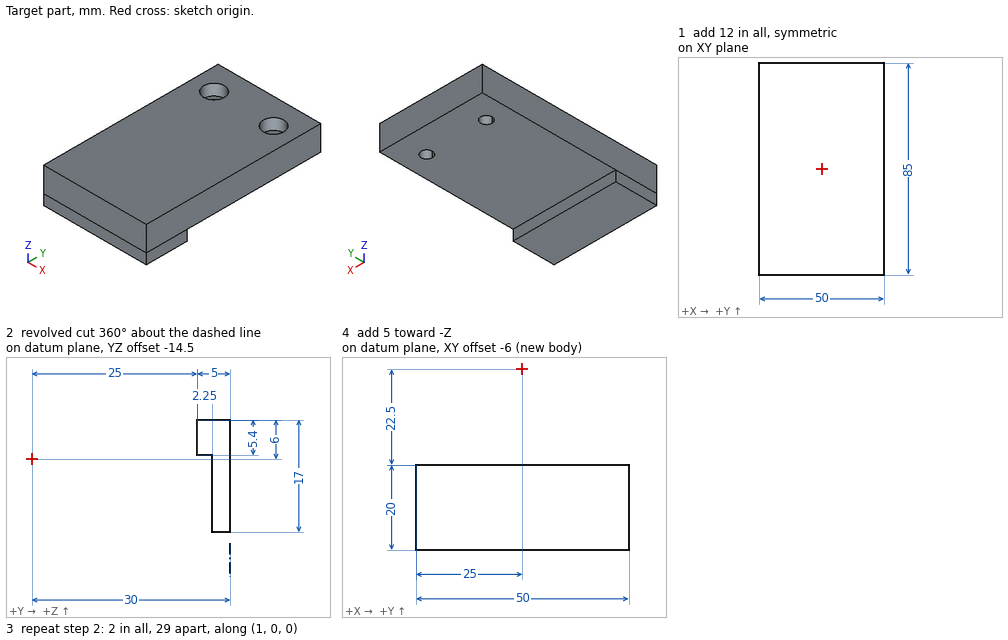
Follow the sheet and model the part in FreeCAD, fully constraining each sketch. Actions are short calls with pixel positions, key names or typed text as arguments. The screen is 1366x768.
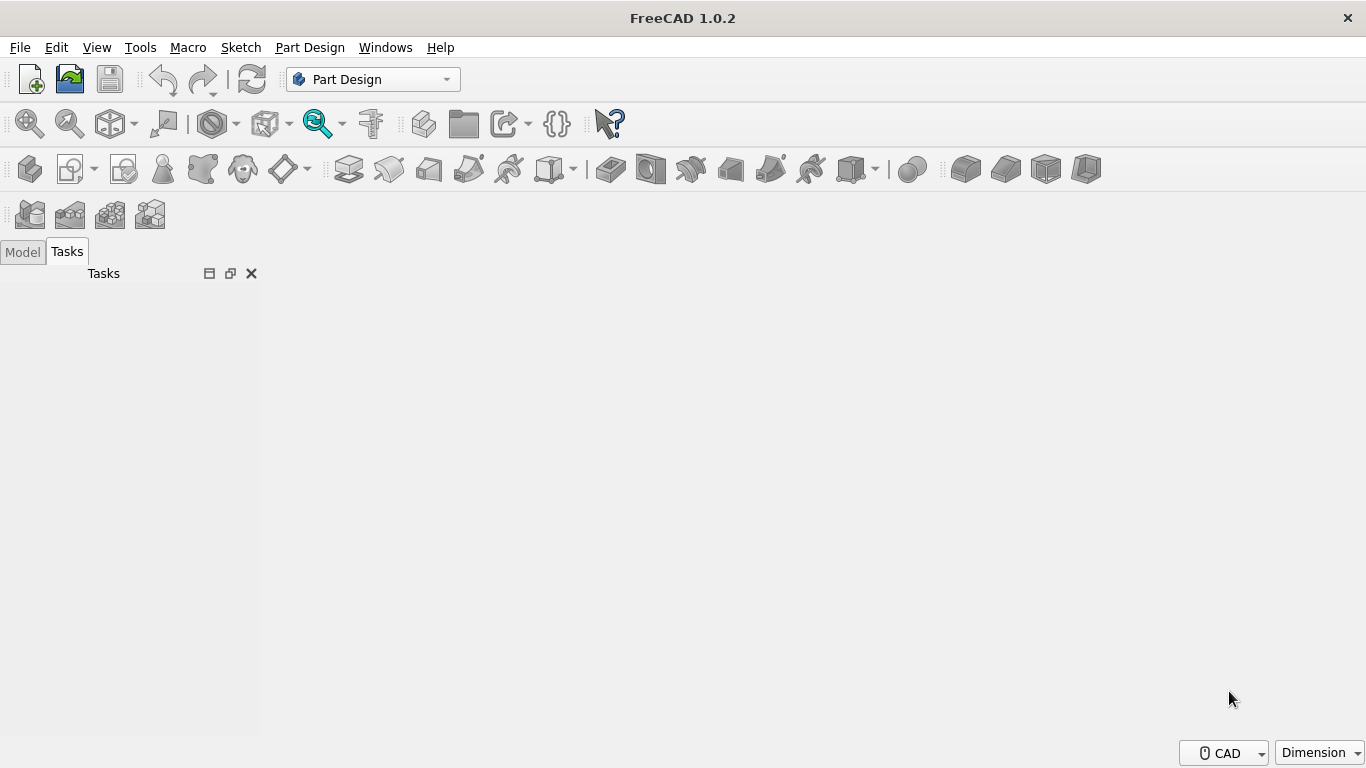
key(ctrl+n)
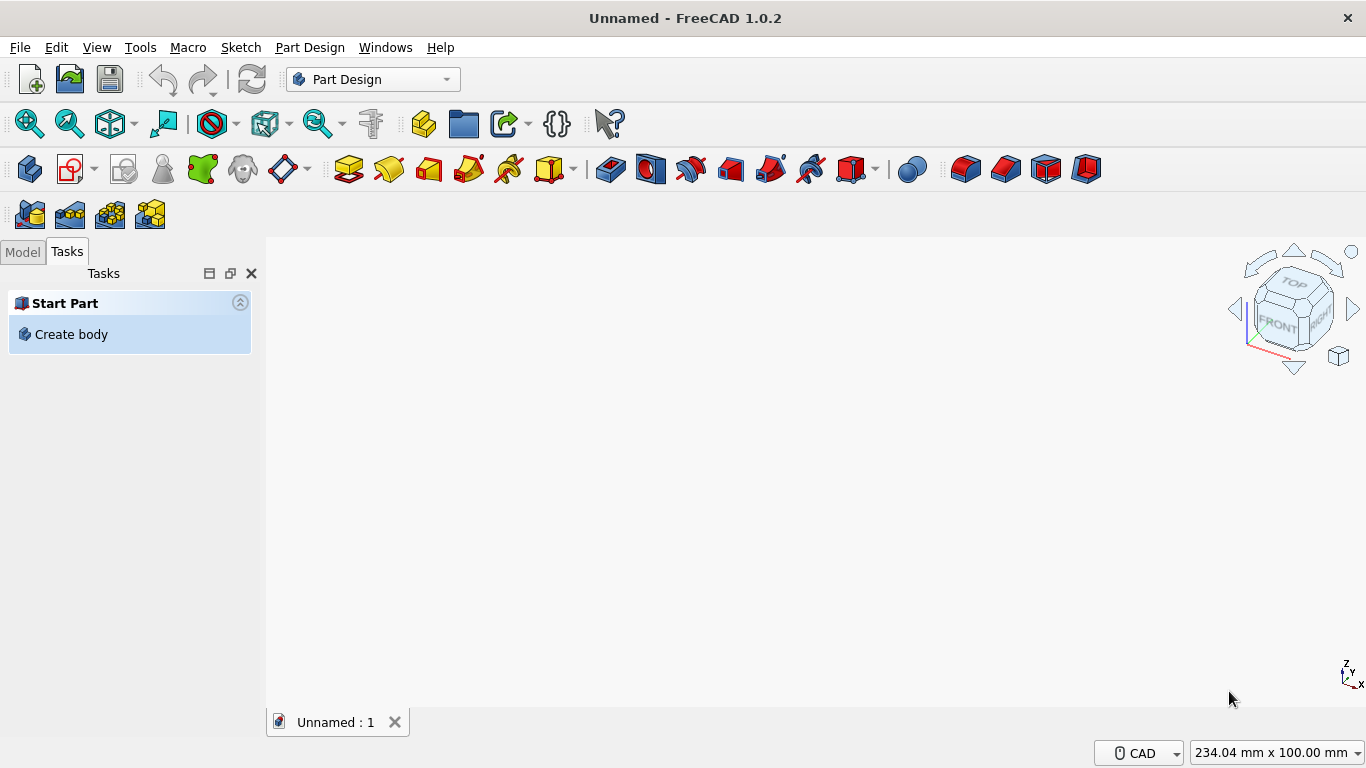
click(70, 170)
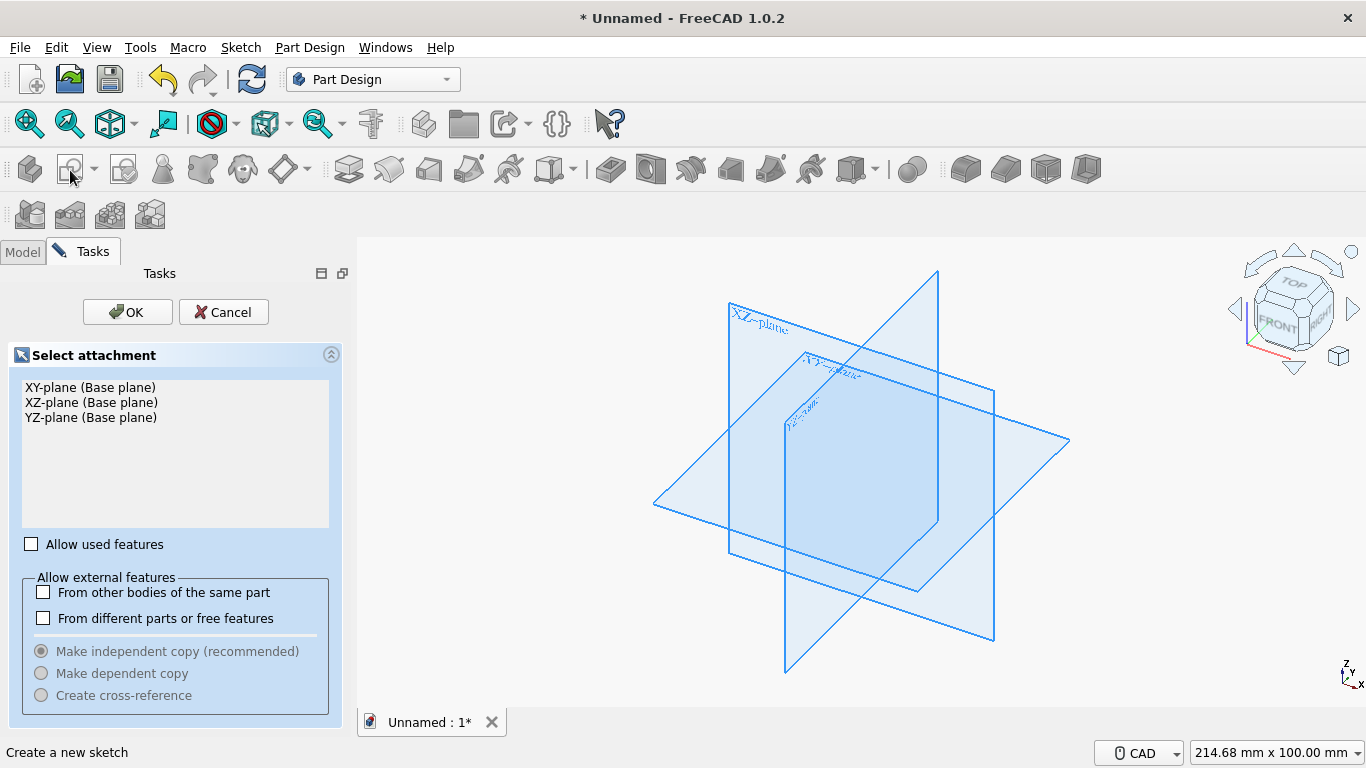
click(82, 388)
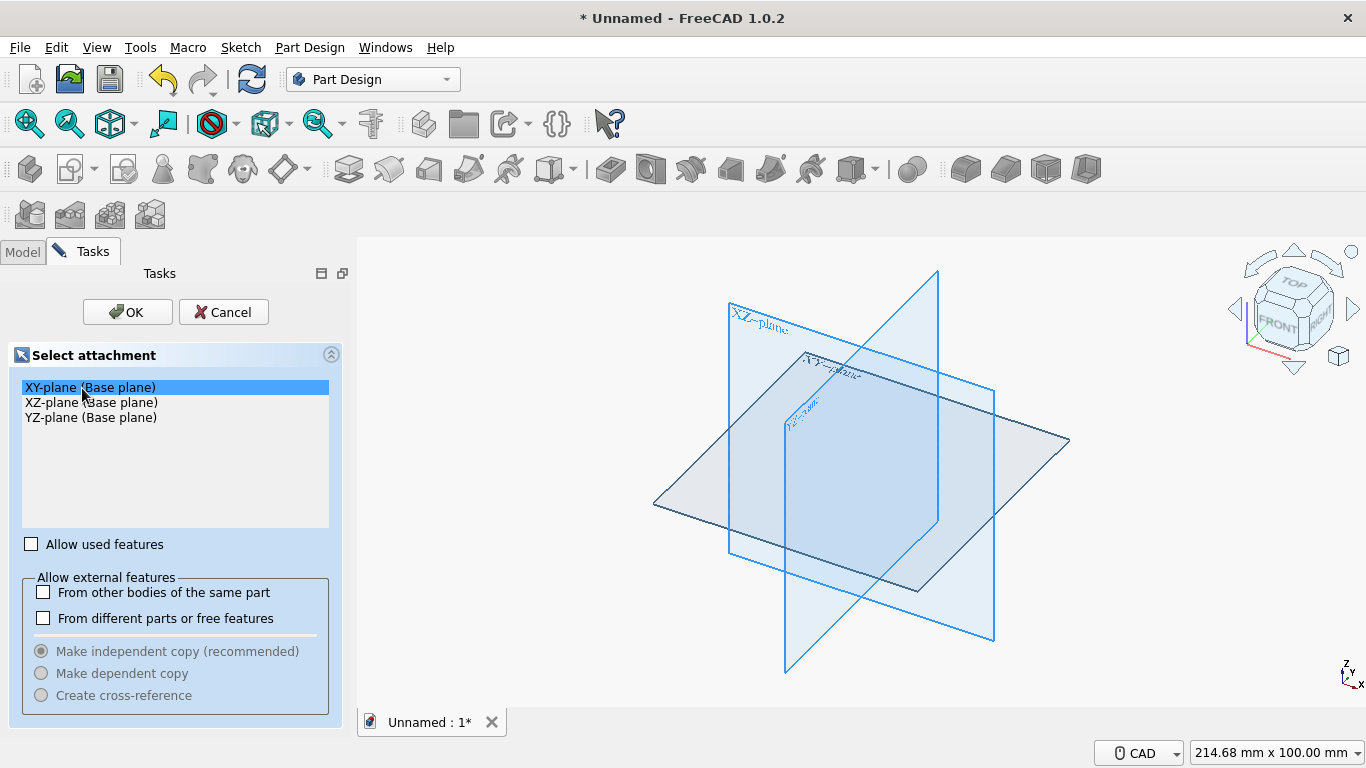
click(128, 312)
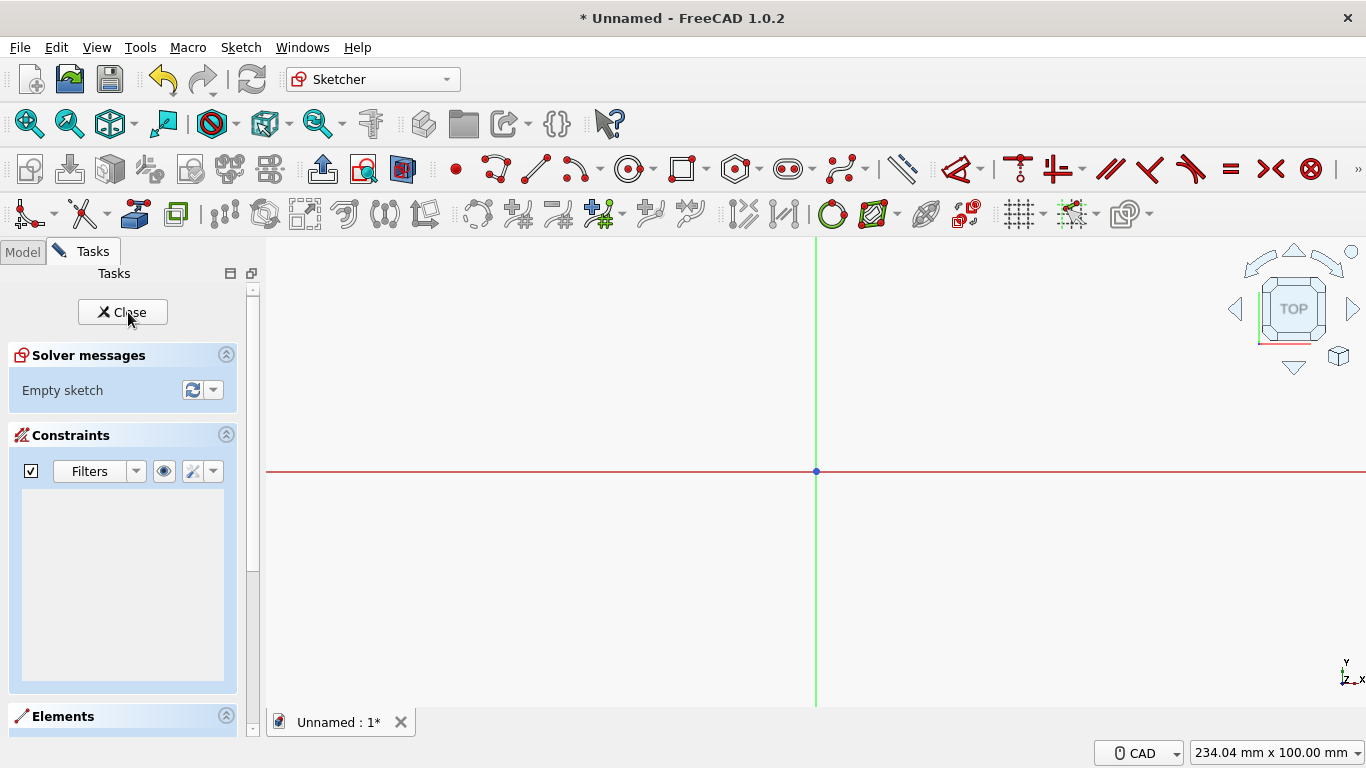
scroll(608, 472, down, 2)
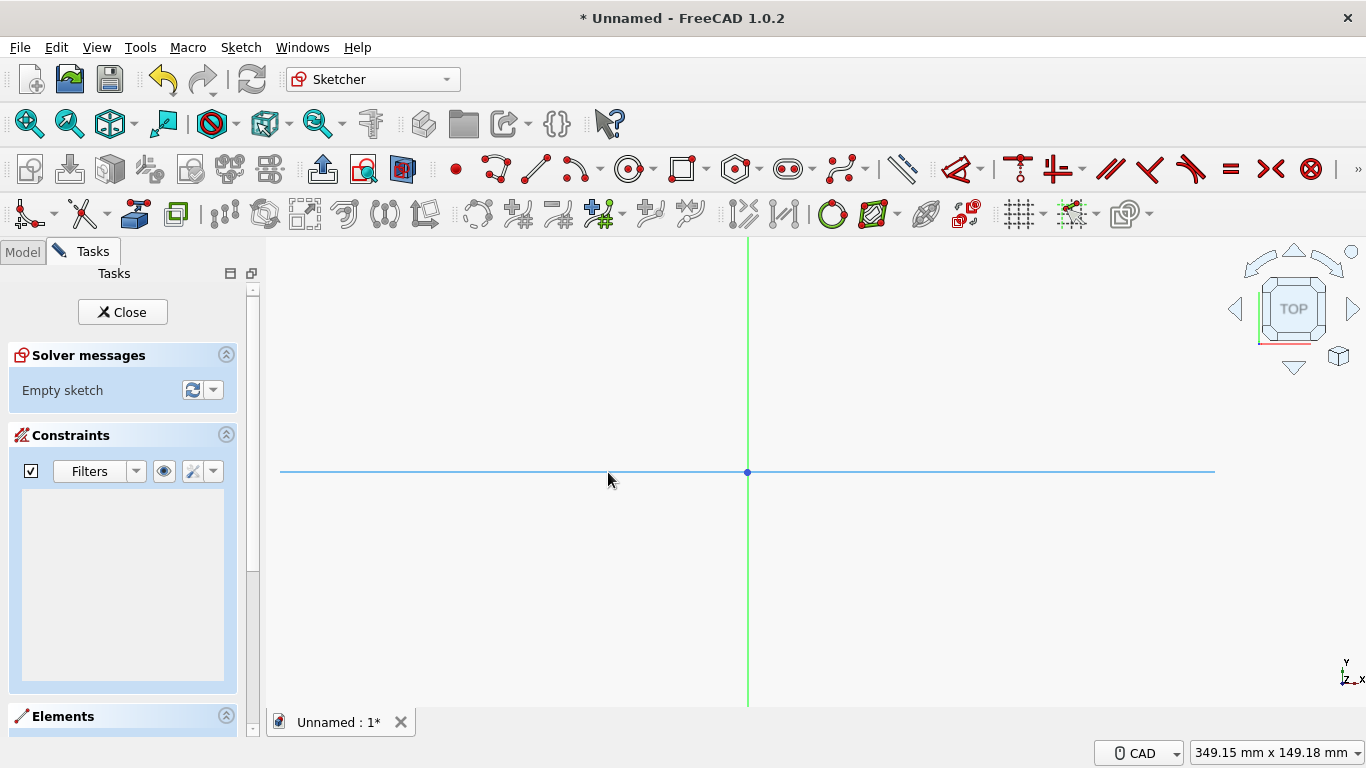
click(708, 170)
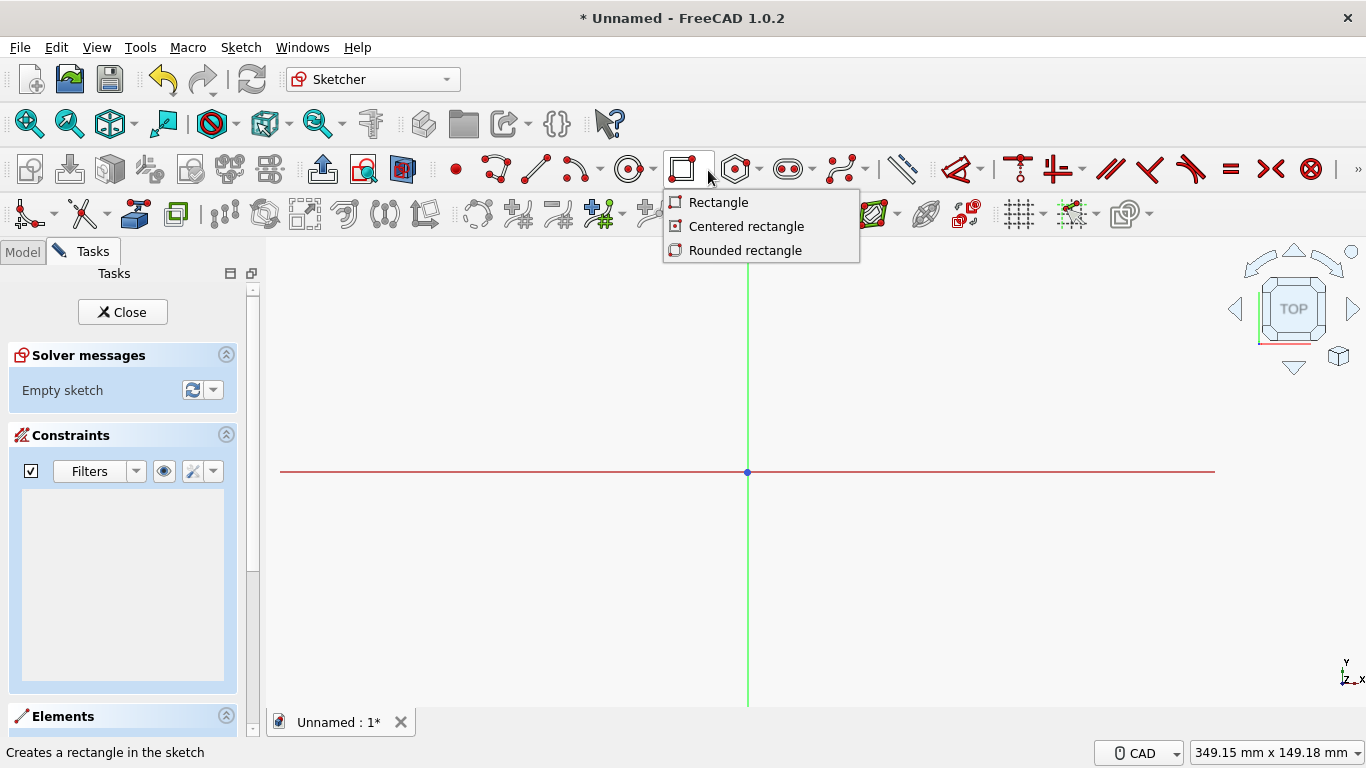
click(762, 226)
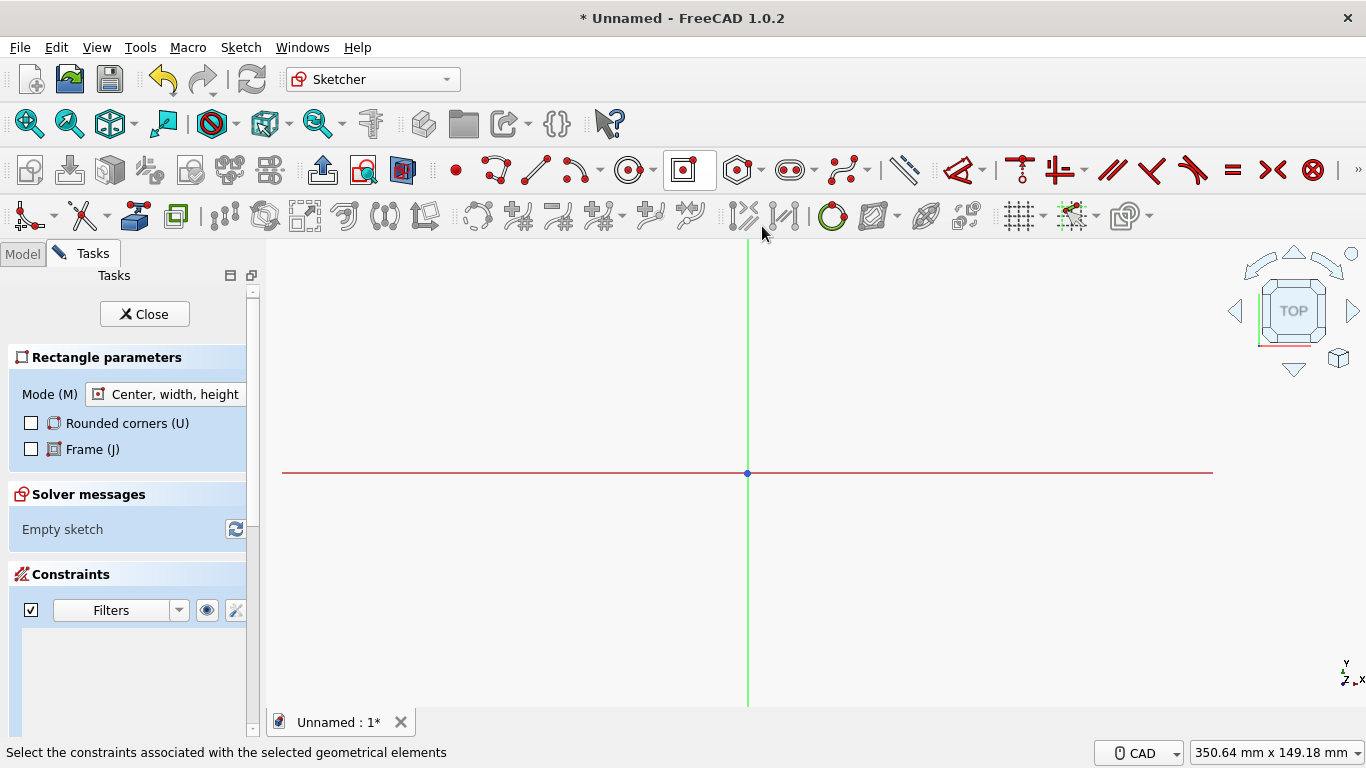
click(748, 473)
click(826, 340)
key(Escape)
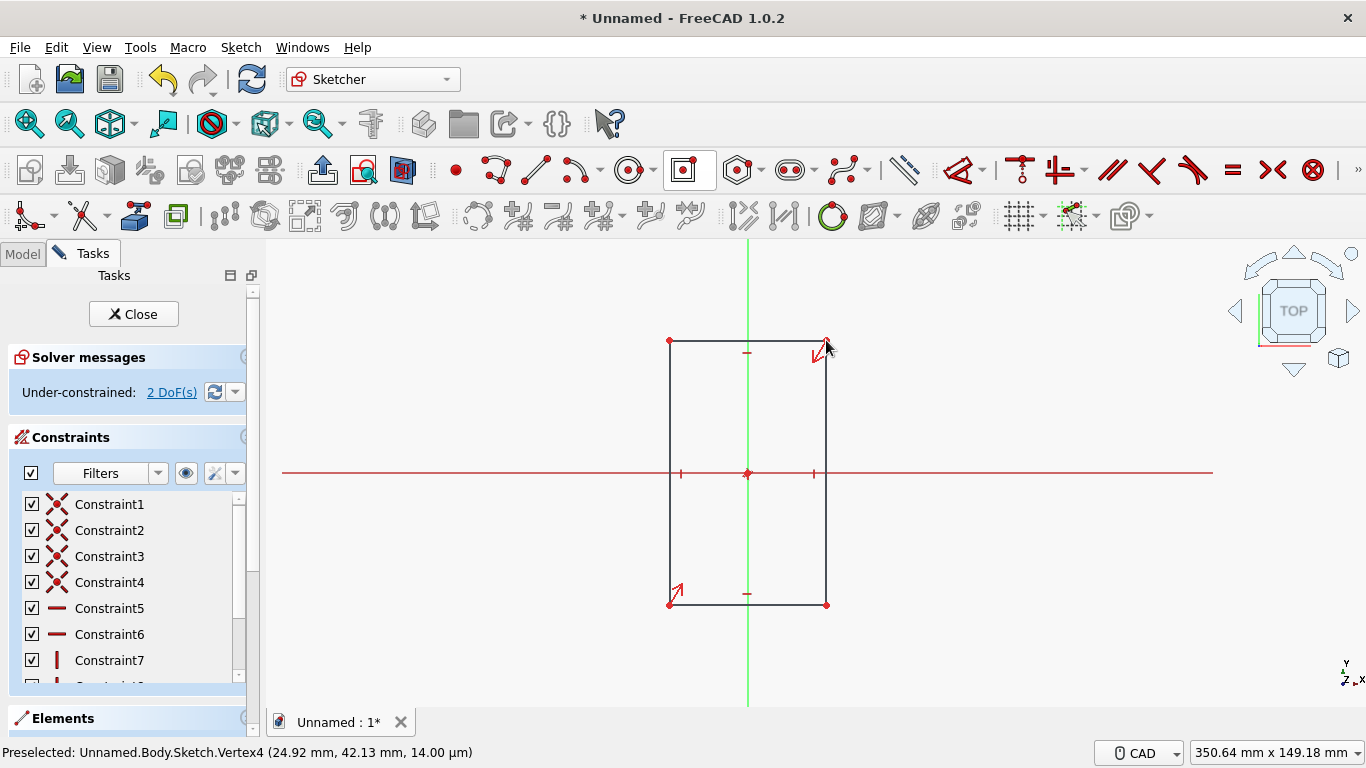
key(d)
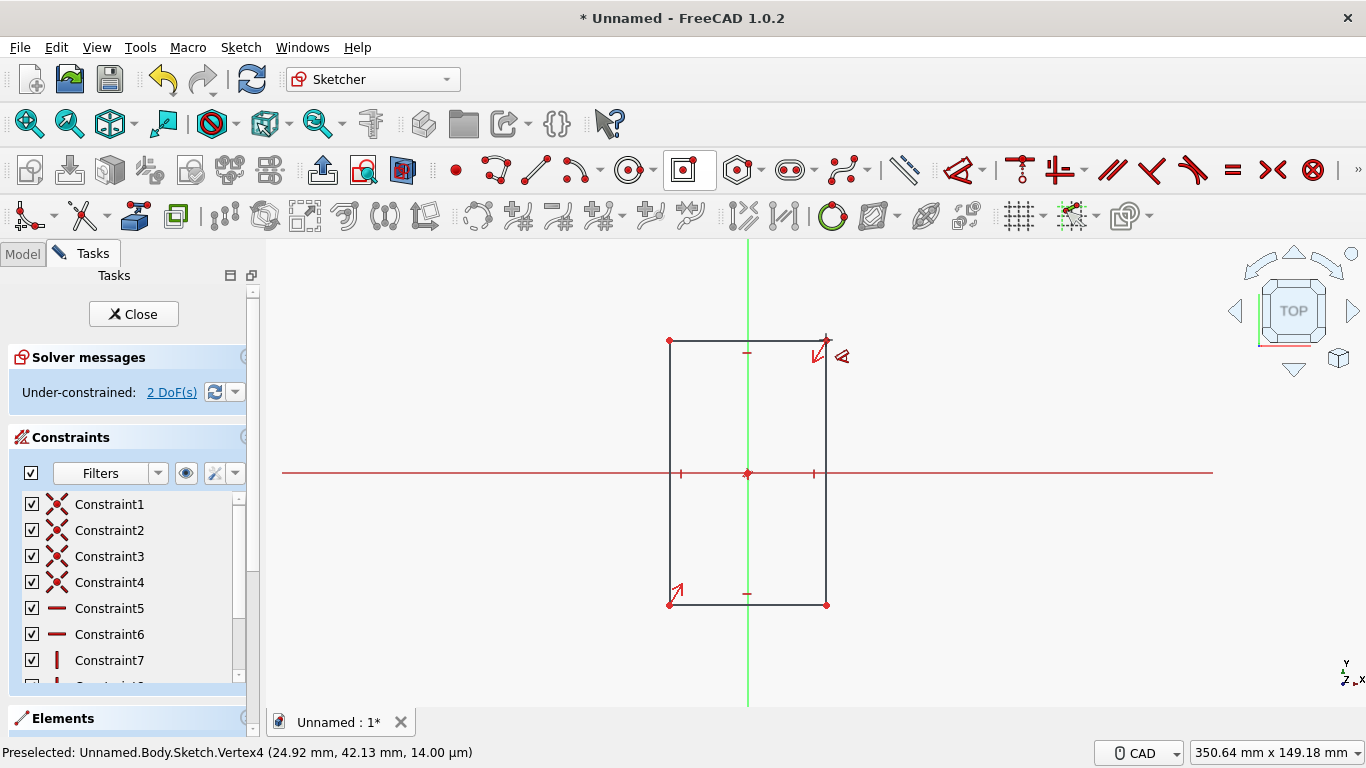
click(717, 605)
click(712, 639)